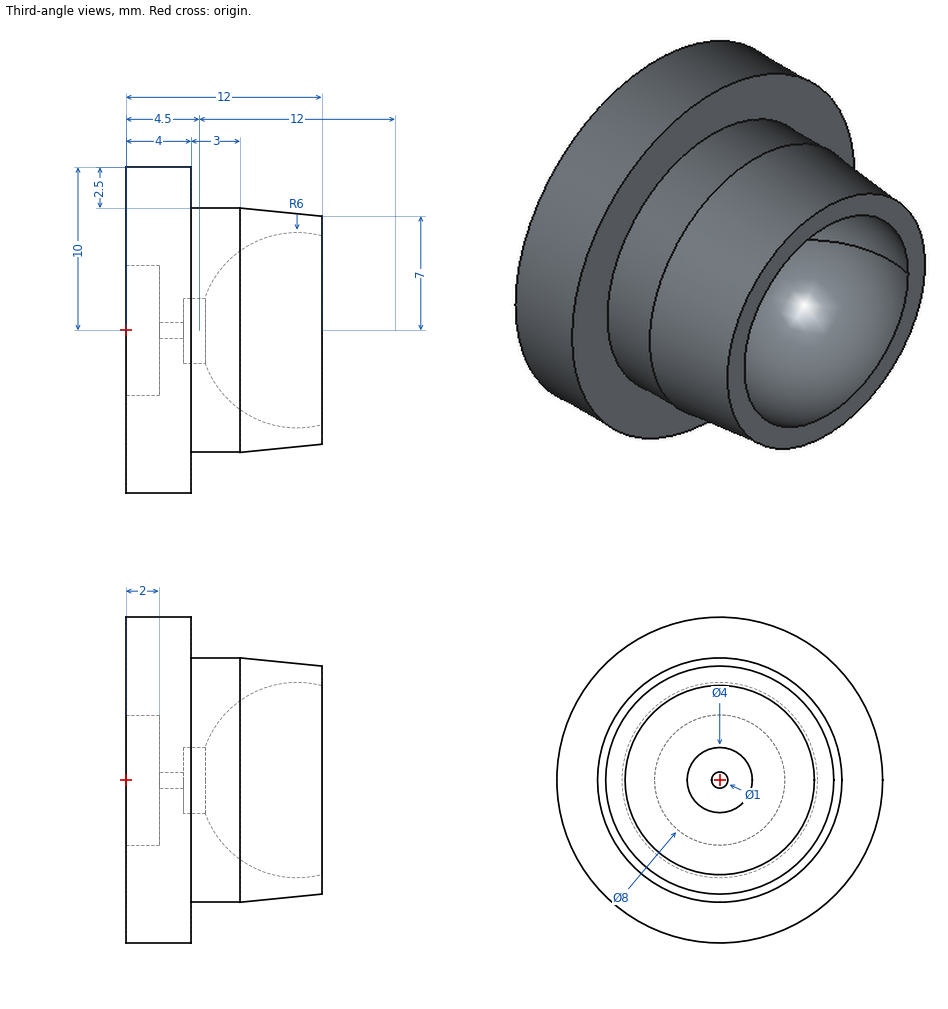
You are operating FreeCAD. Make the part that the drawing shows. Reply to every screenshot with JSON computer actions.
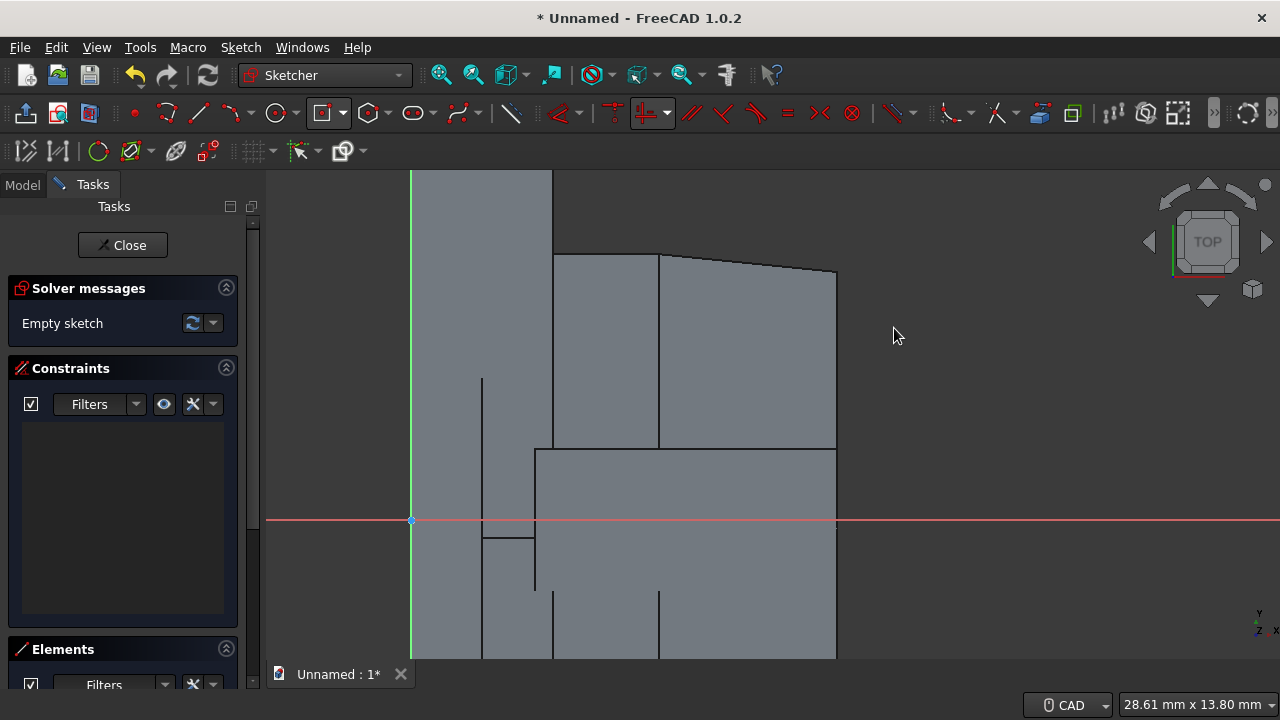
{"action": "left_click", "coordinate": [200, 114]}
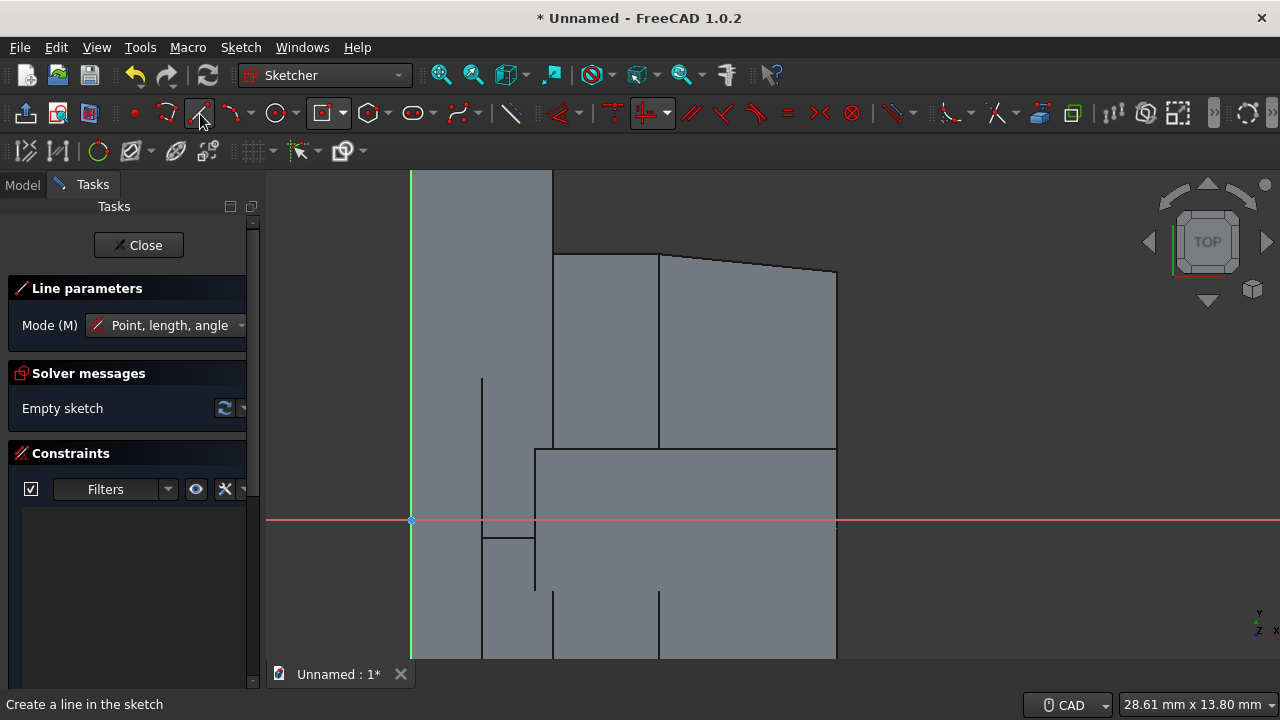
{"action": "left_click", "coordinate": [571, 520]}
{"action": "left_click", "coordinate": [996, 511]}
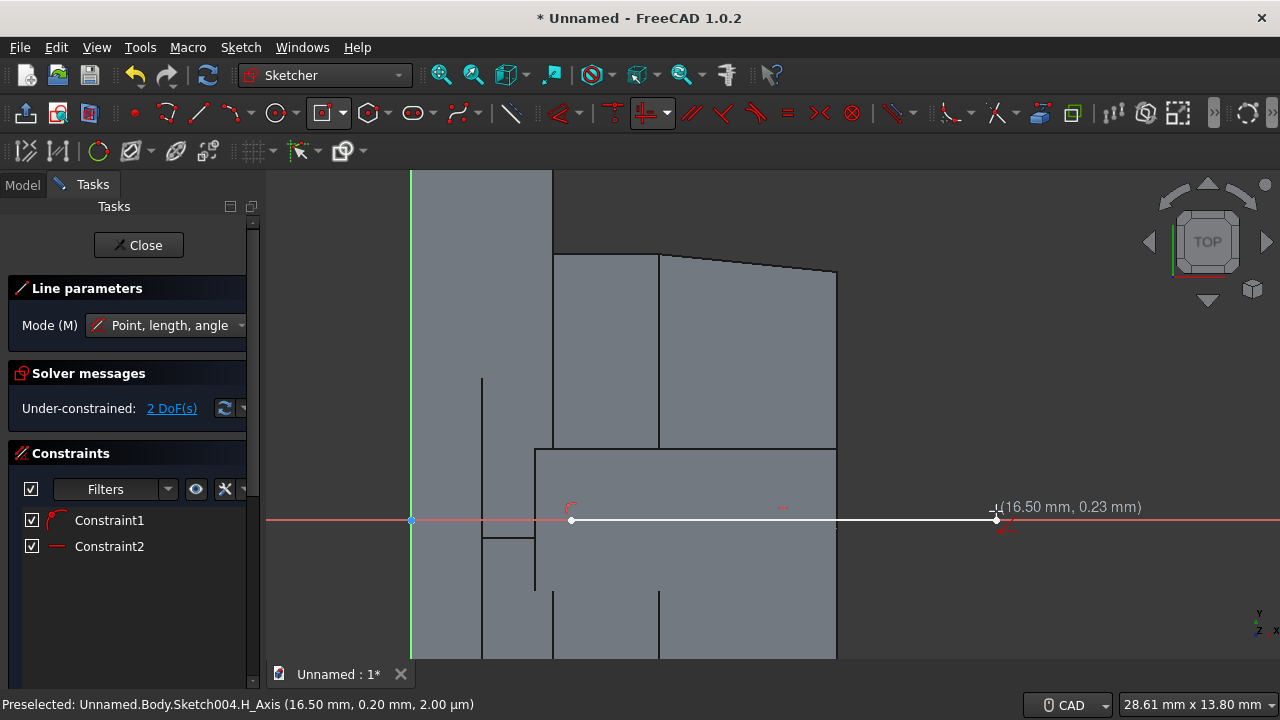
{"action": "left_click", "coordinate": [232, 114]}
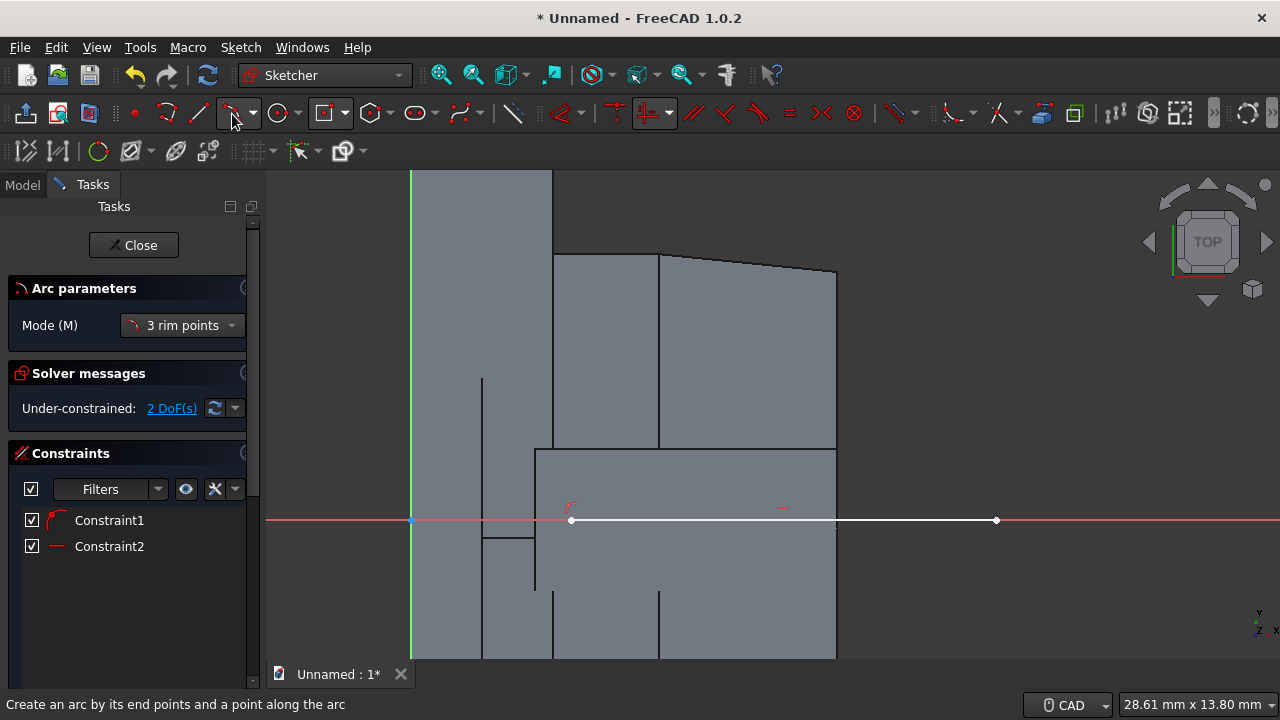
{"action": "left_click", "coordinate": [996, 511]}
{"action": "left_click", "coordinate": [571, 520]}
{"action": "left_click", "coordinate": [783, 307]}
{"action": "key", "text": "Escape"}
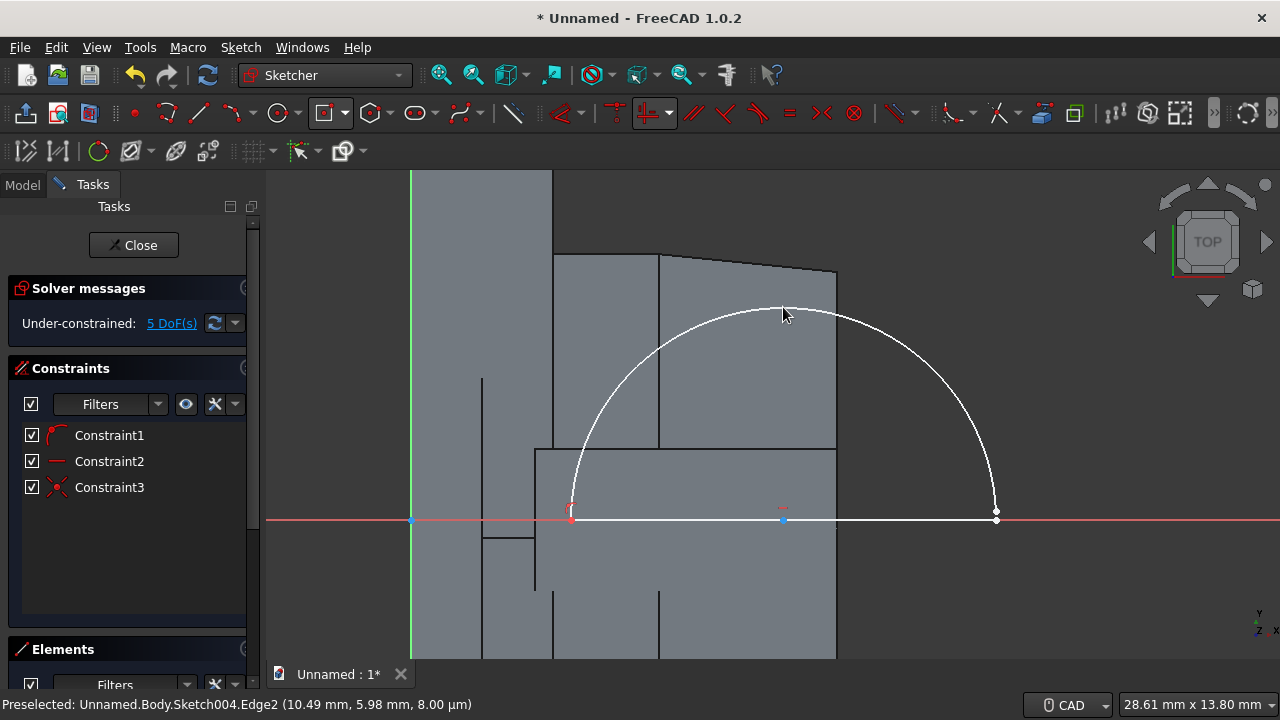
{"action": "left_click", "coordinate": [784, 521]}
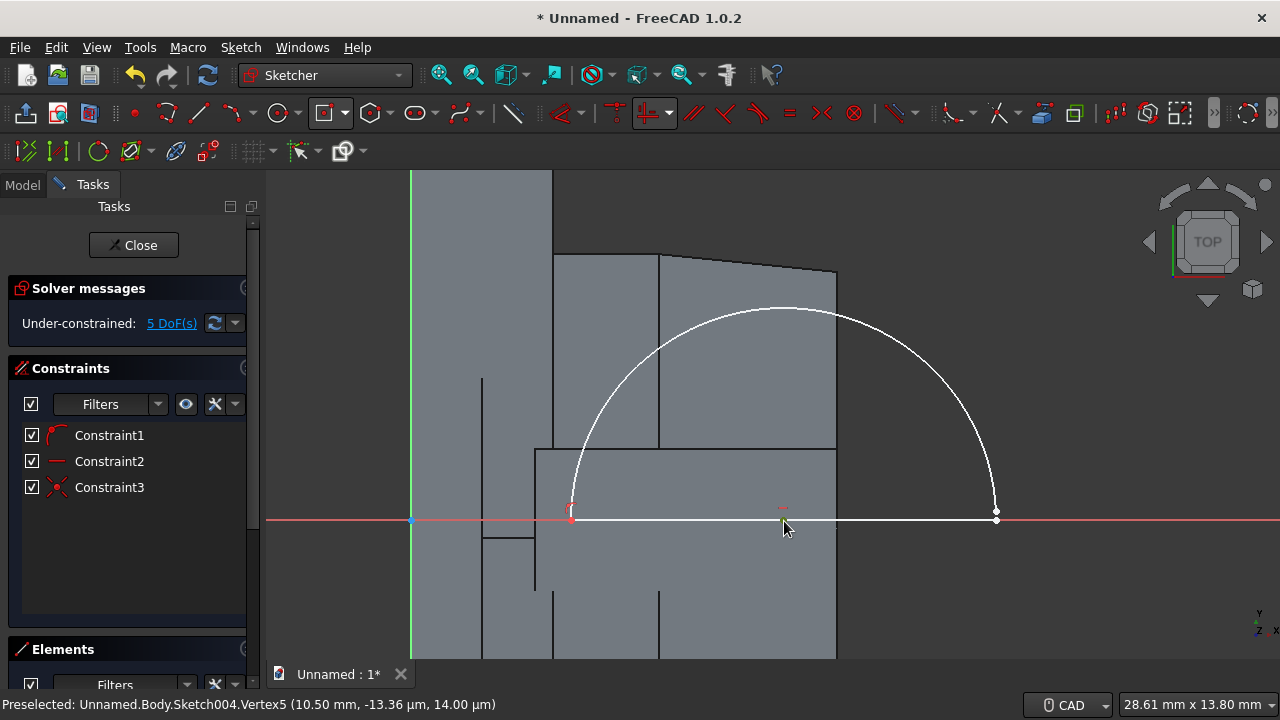
{"action": "left_click", "coordinate": [353, 520]}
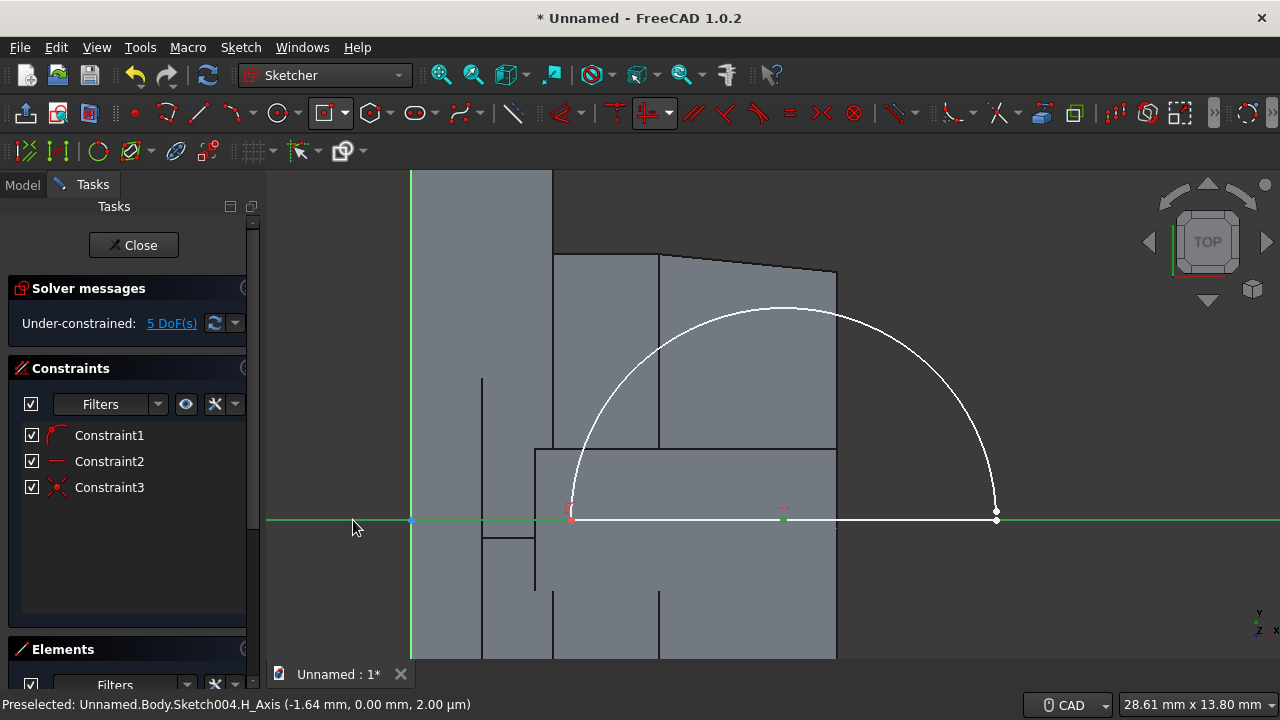
{"action": "left_click", "coordinate": [616, 114]}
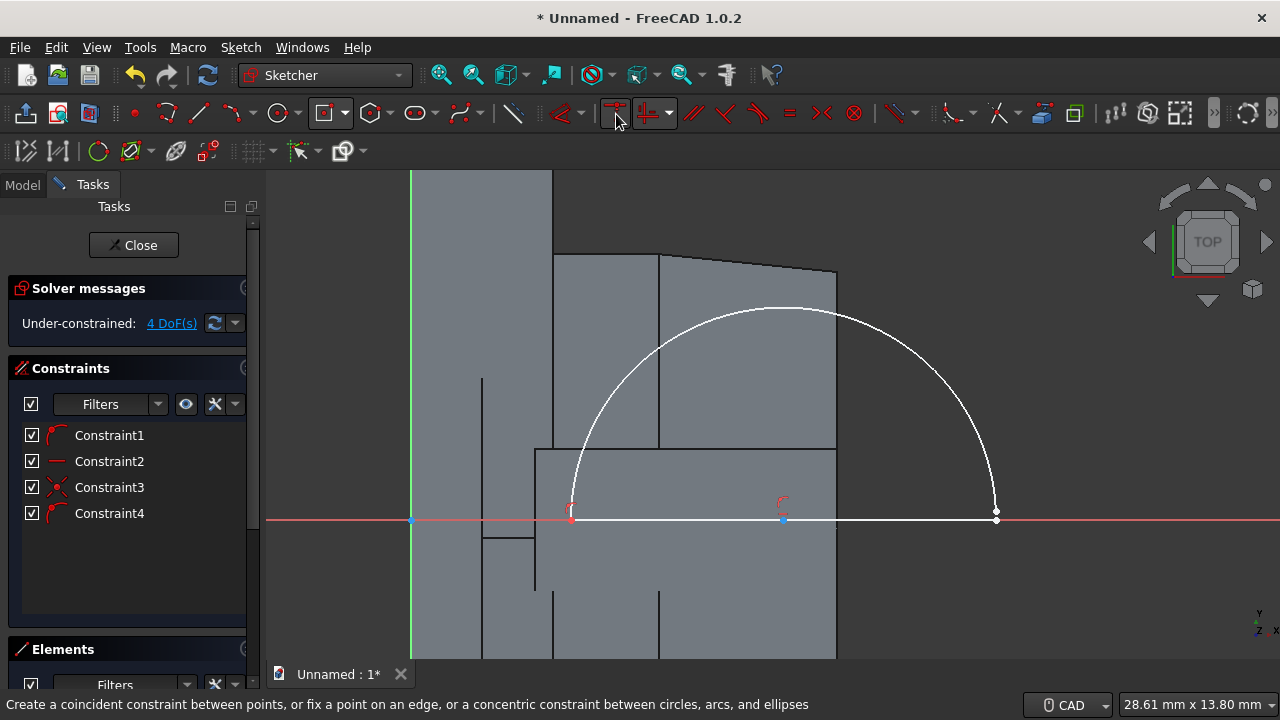
{"action": "left_click", "coordinate": [560, 114]}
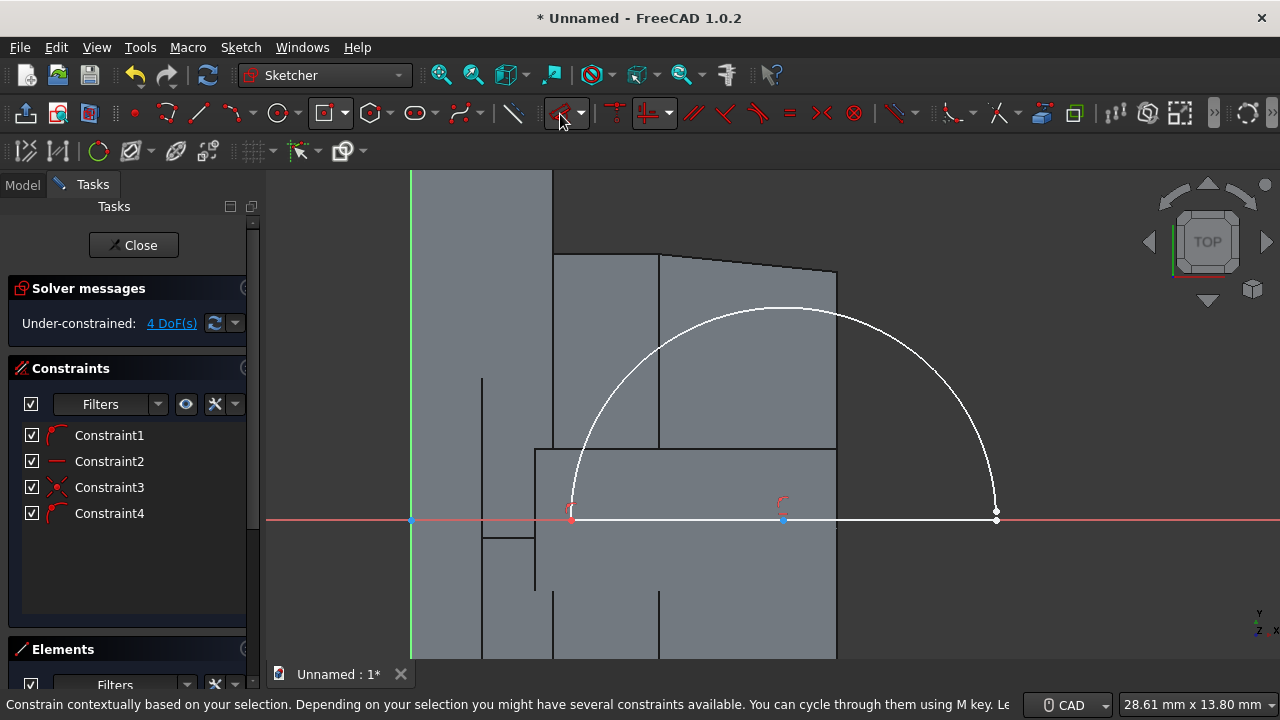
{"action": "left_click", "coordinate": [904, 345]}
{"action": "left_click", "coordinate": [922, 319]}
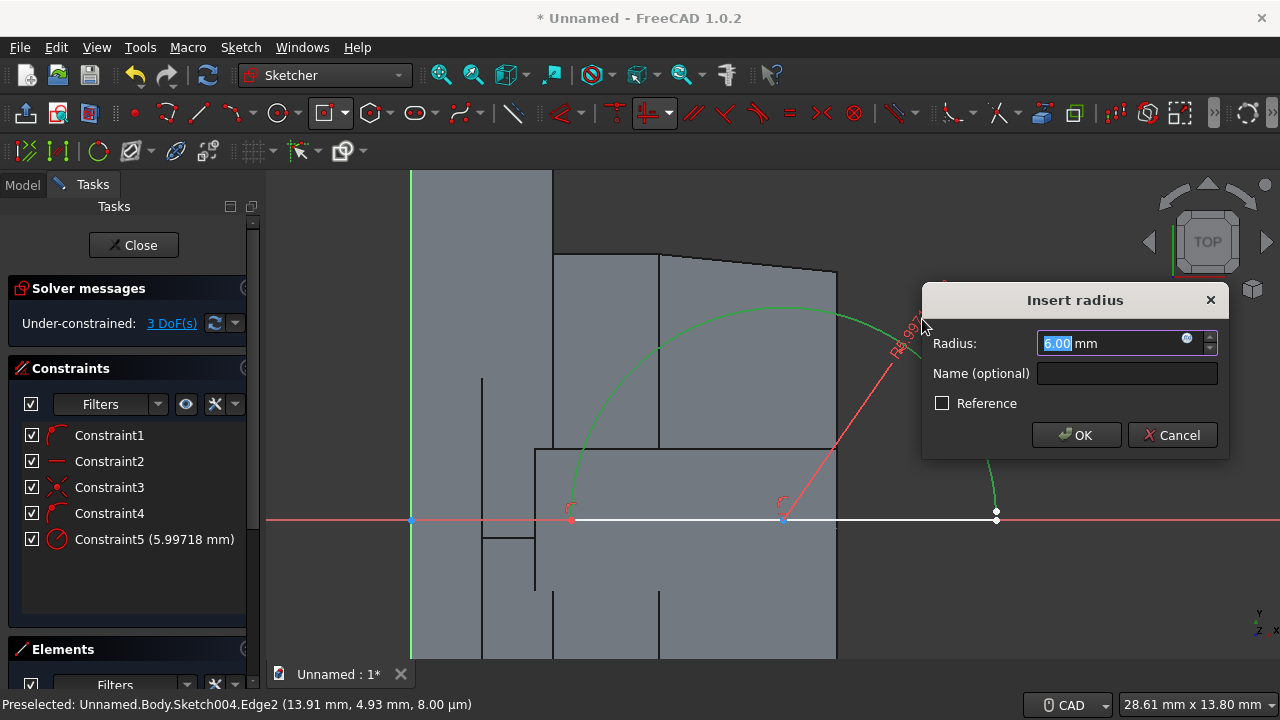
{"action": "type", "text": "6"}
{"action": "key", "text": "Return"}
{"action": "key", "text": "Escape"}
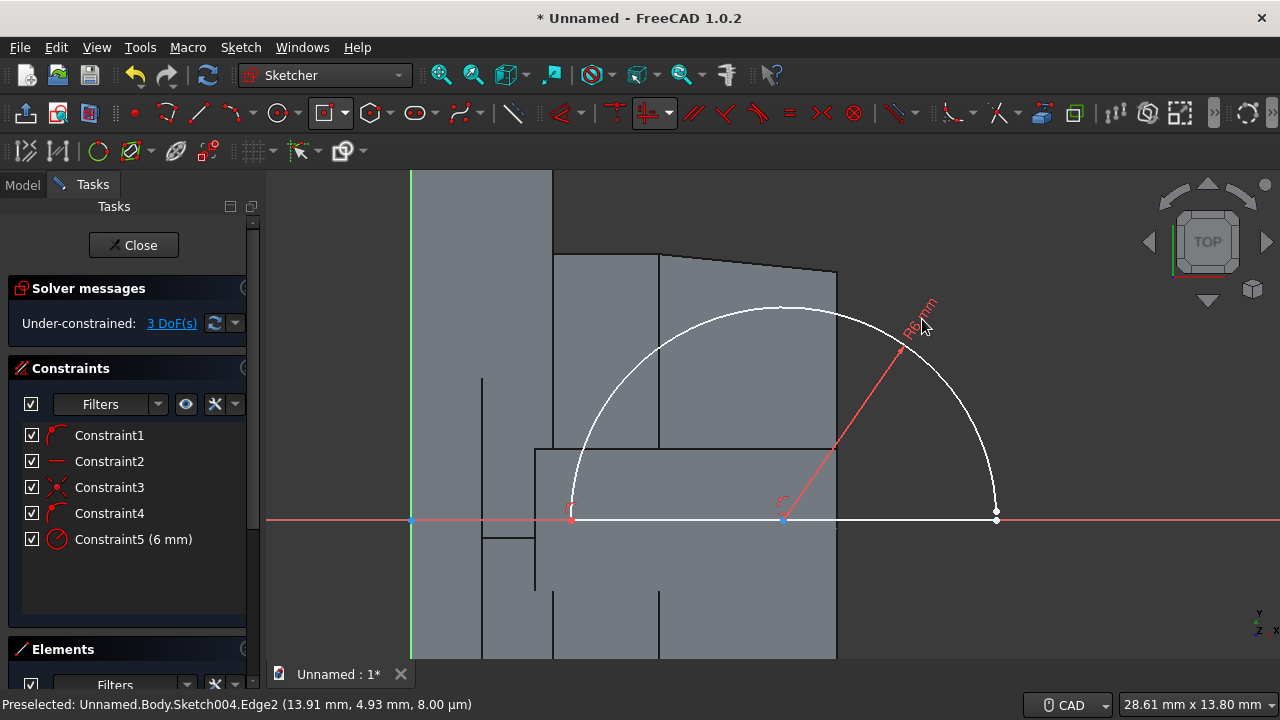
{"action": "left_click", "coordinate": [996, 512]}